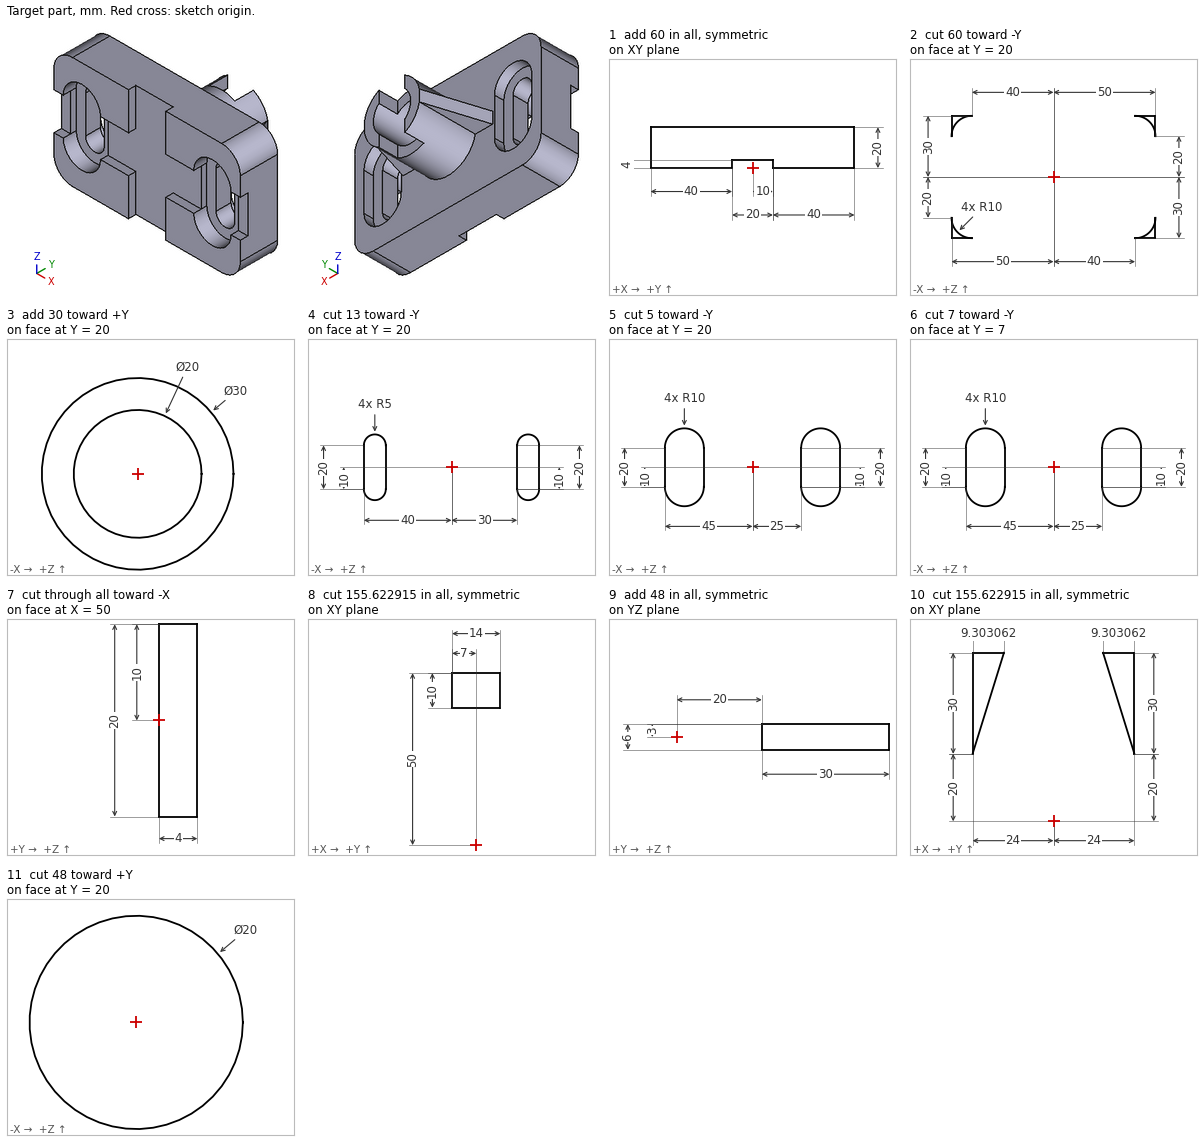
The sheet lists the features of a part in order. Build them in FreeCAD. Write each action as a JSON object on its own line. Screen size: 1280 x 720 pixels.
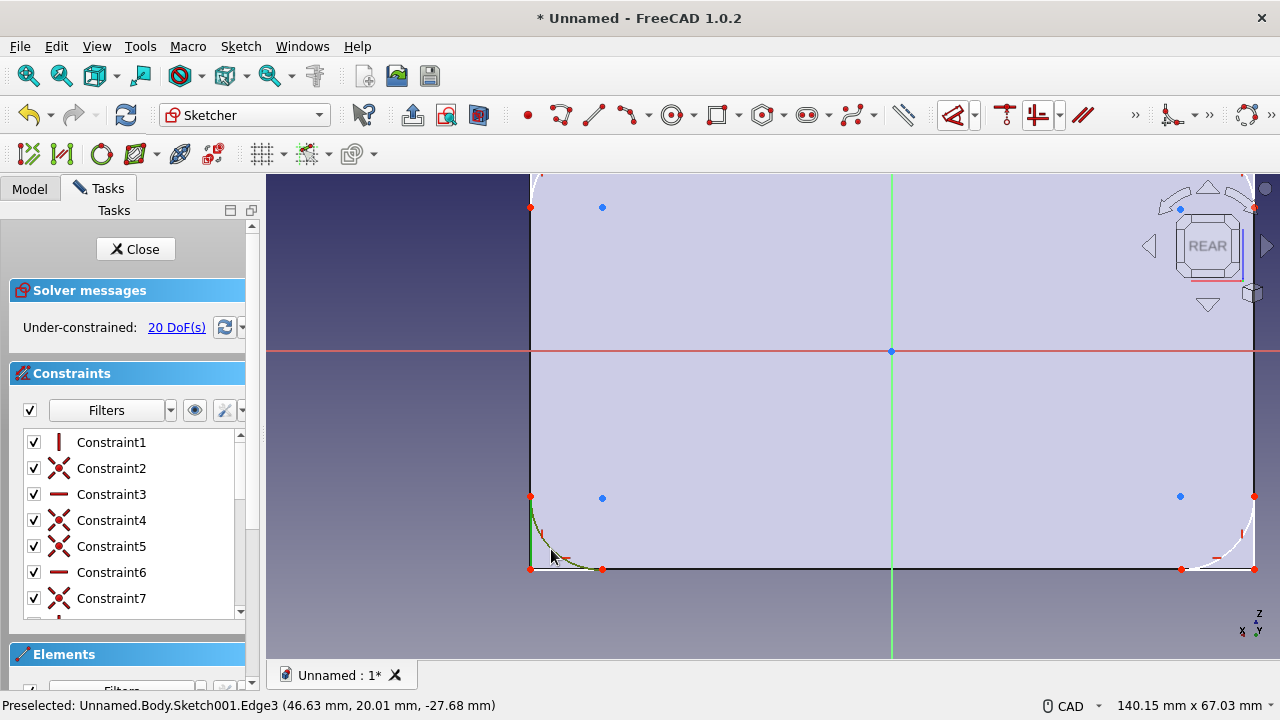
{"action": "key", "text": "t"}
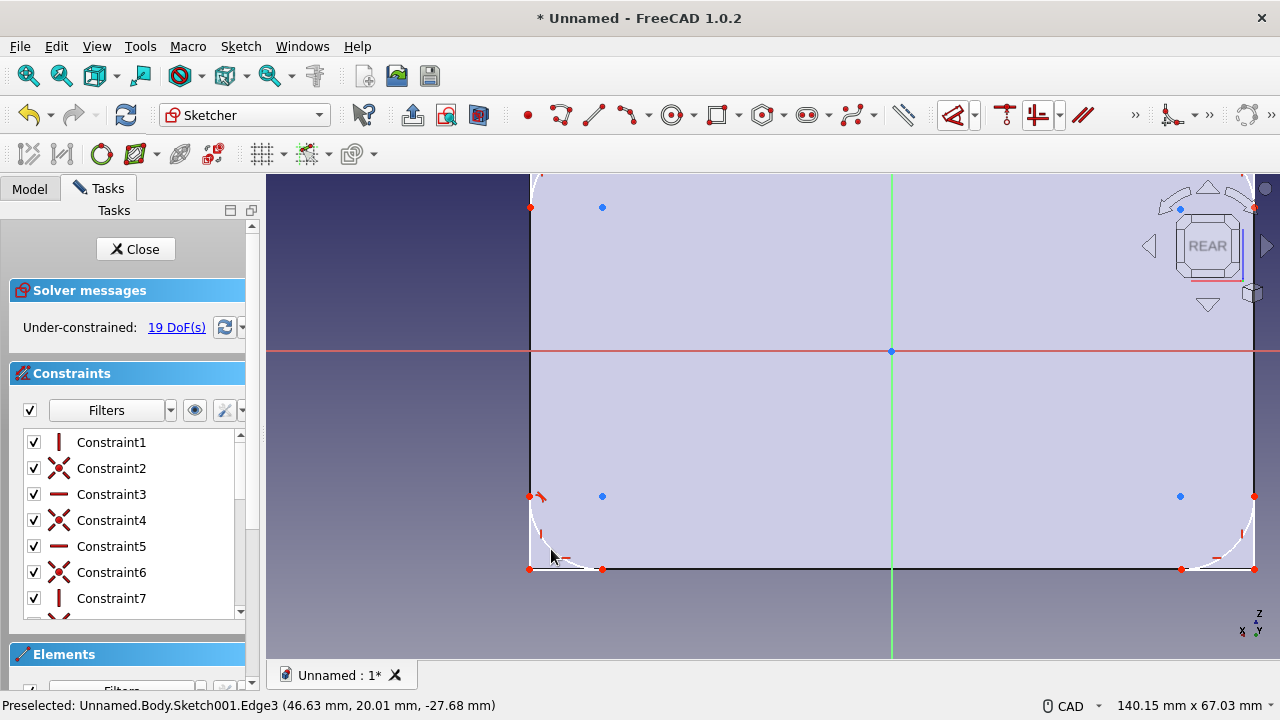
{"action": "left_click", "coordinate": [551, 570]}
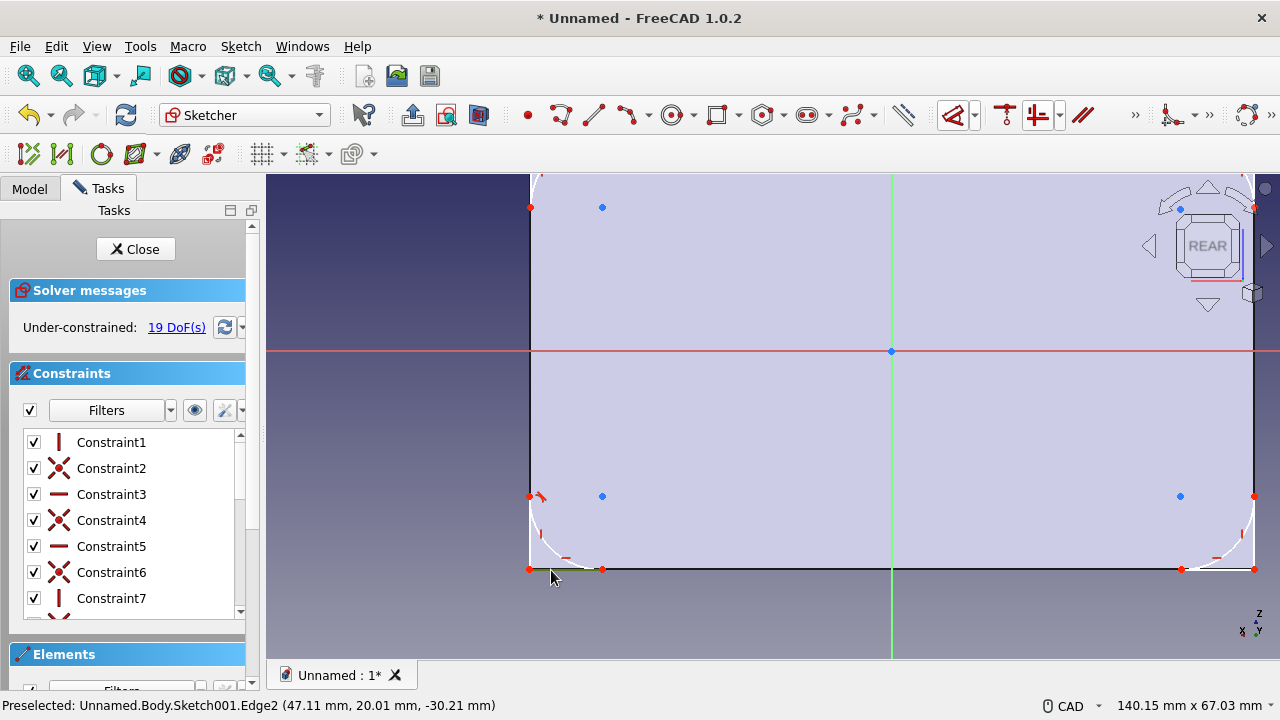
{"action": "left_click", "coordinate": [551, 549]}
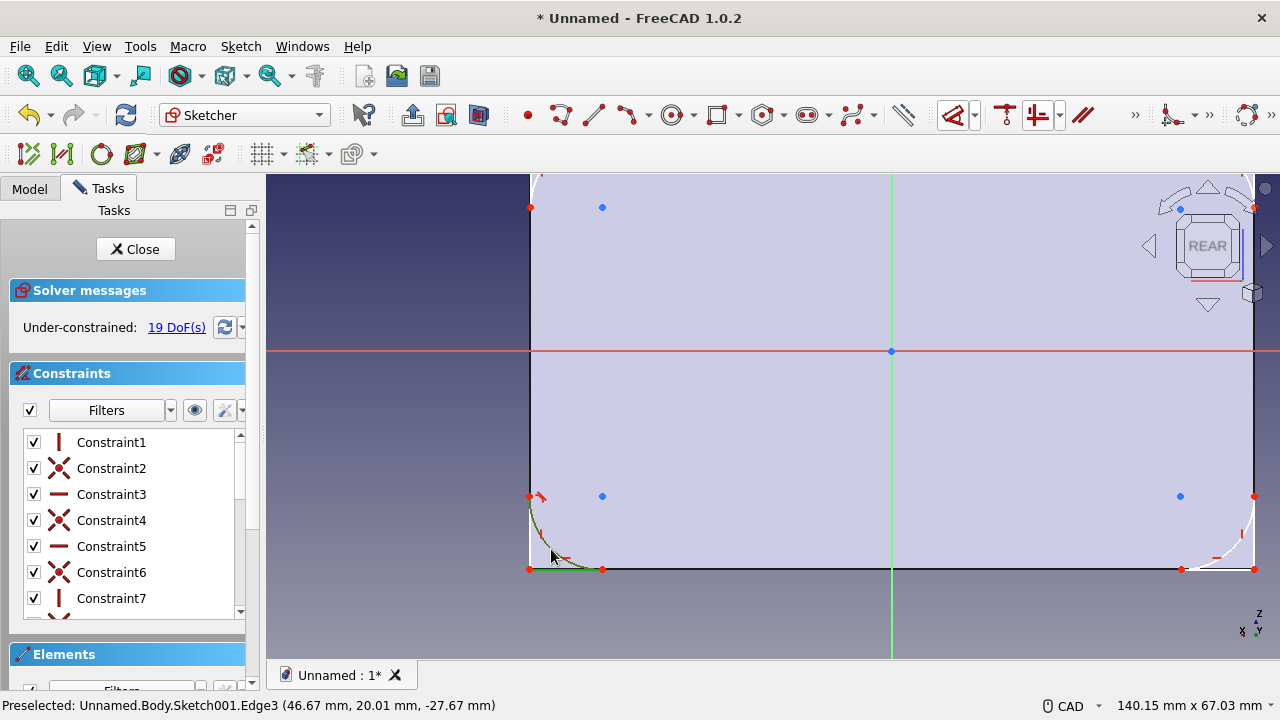
{"action": "key", "text": "t"}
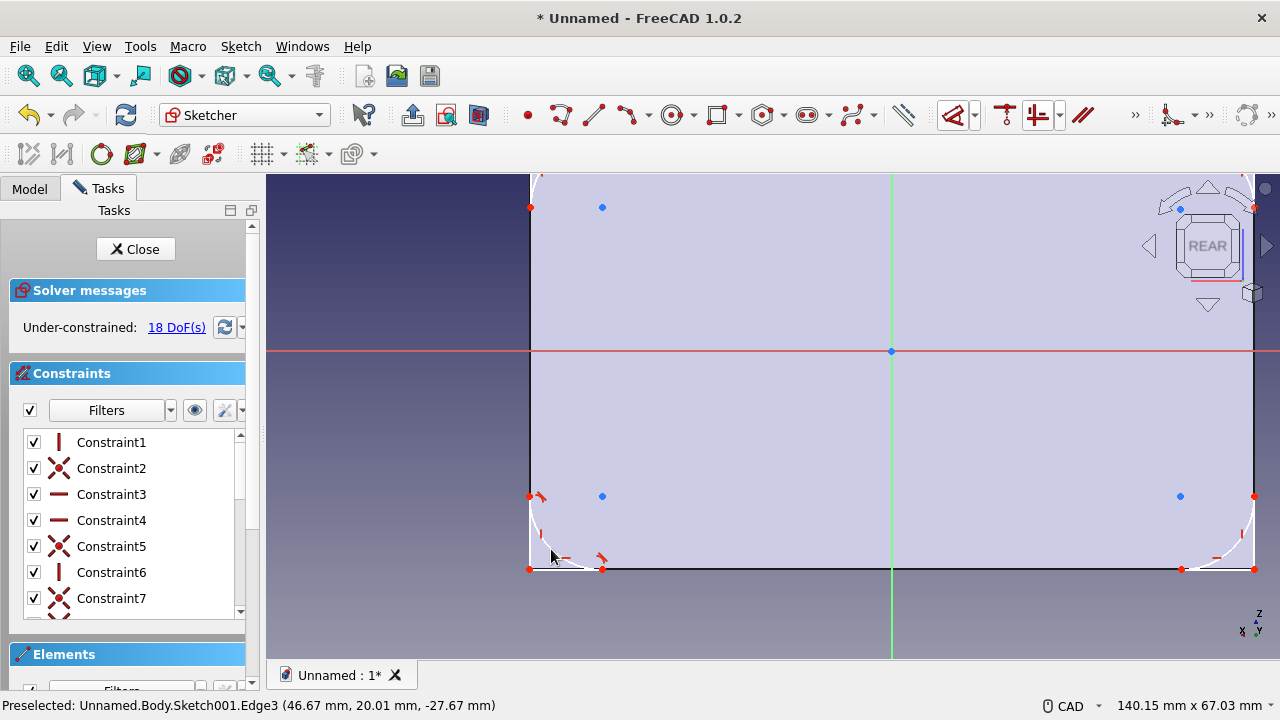
{"action": "scroll", "coordinate": [323, 549], "scroll_direction": "down", "scroll_amount": 2}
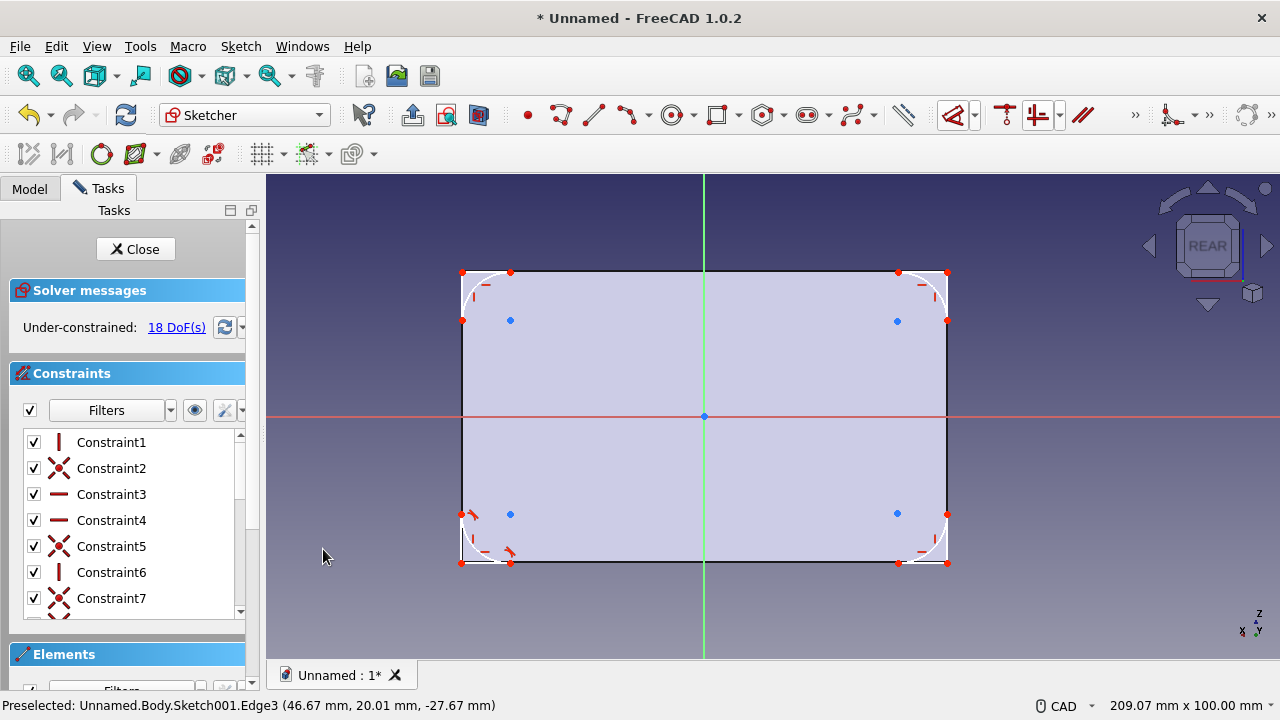
{"action": "scroll", "coordinate": [933, 563], "scroll_direction": "up", "scroll_amount": 2}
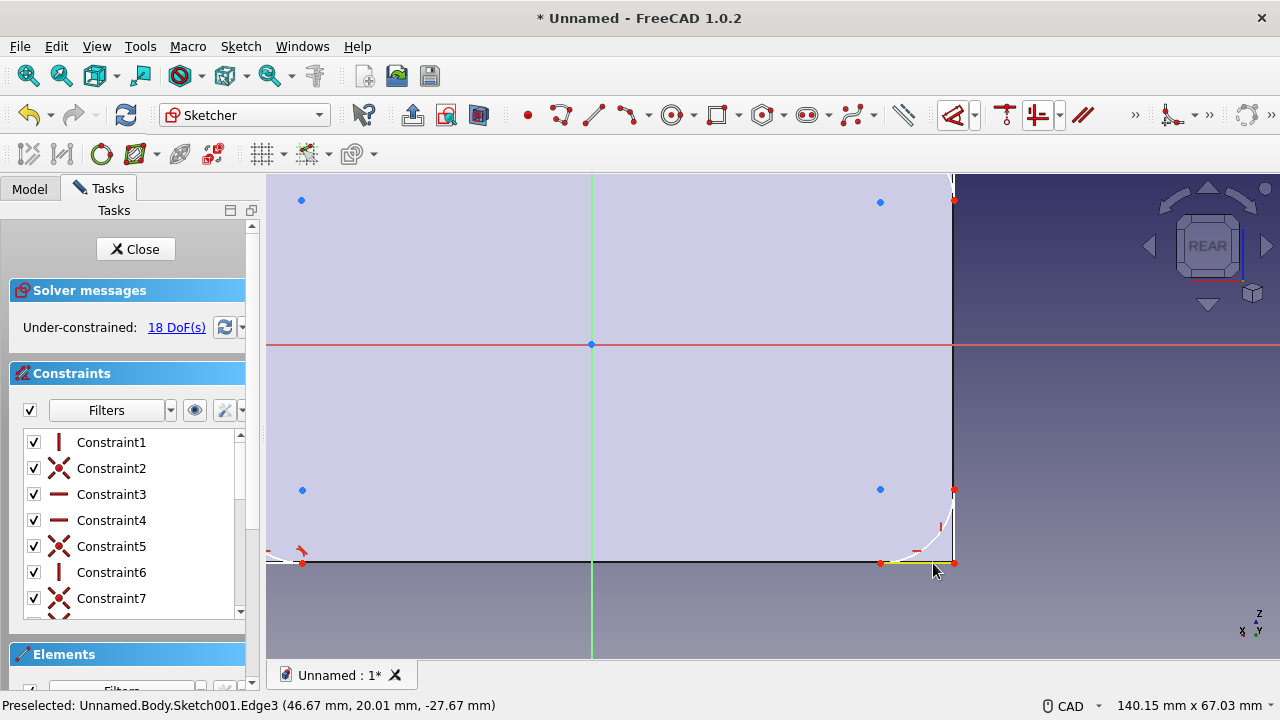
{"action": "left_click", "coordinate": [932, 563]}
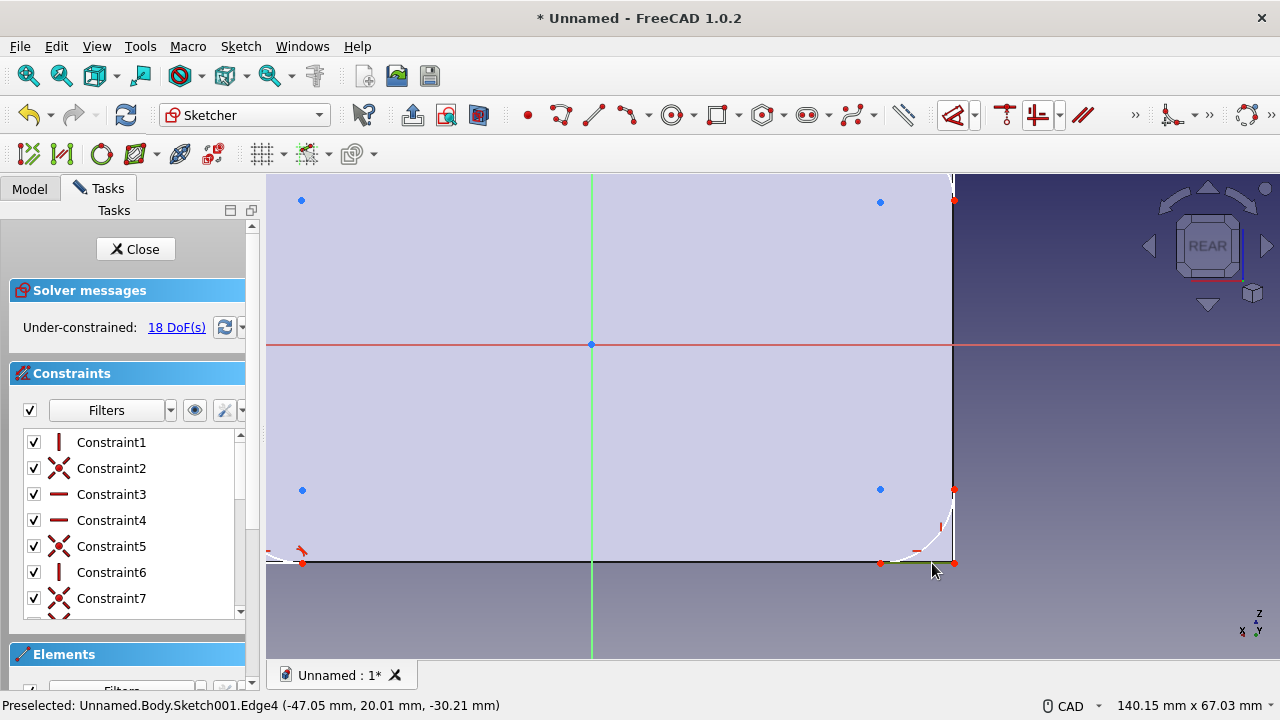
{"action": "left_click", "coordinate": [932, 541]}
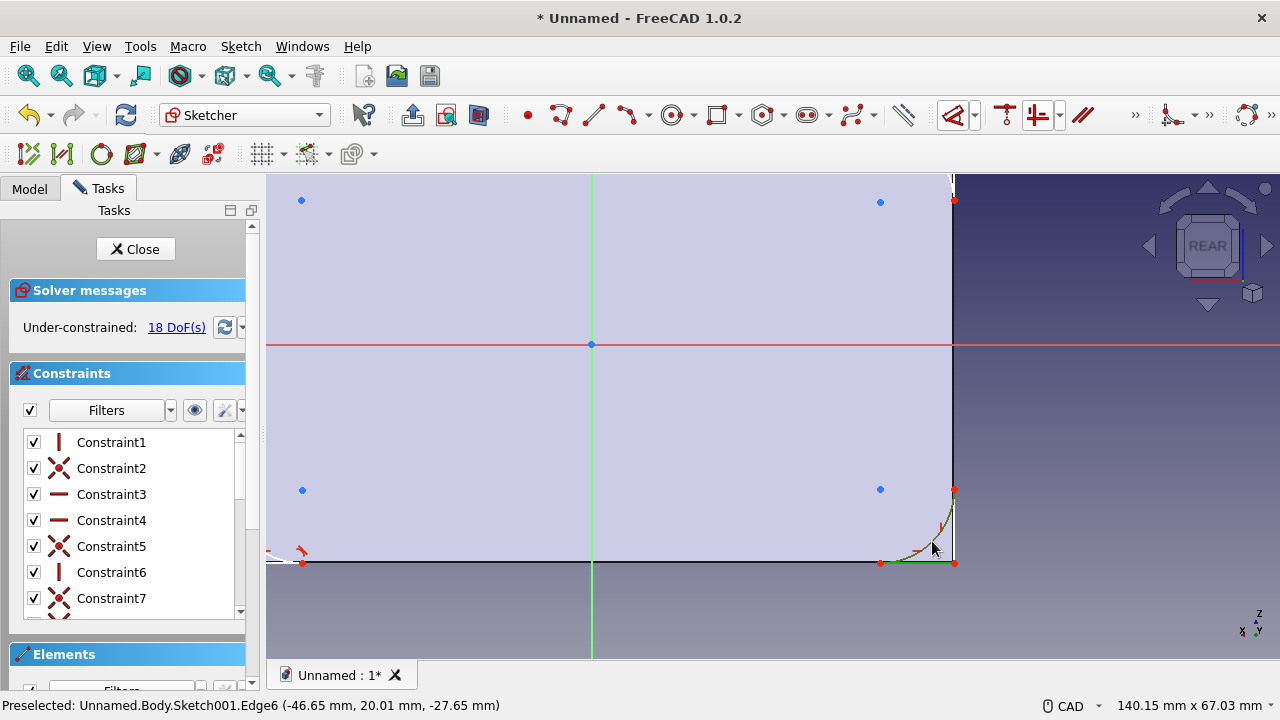
{"action": "key", "text": "t"}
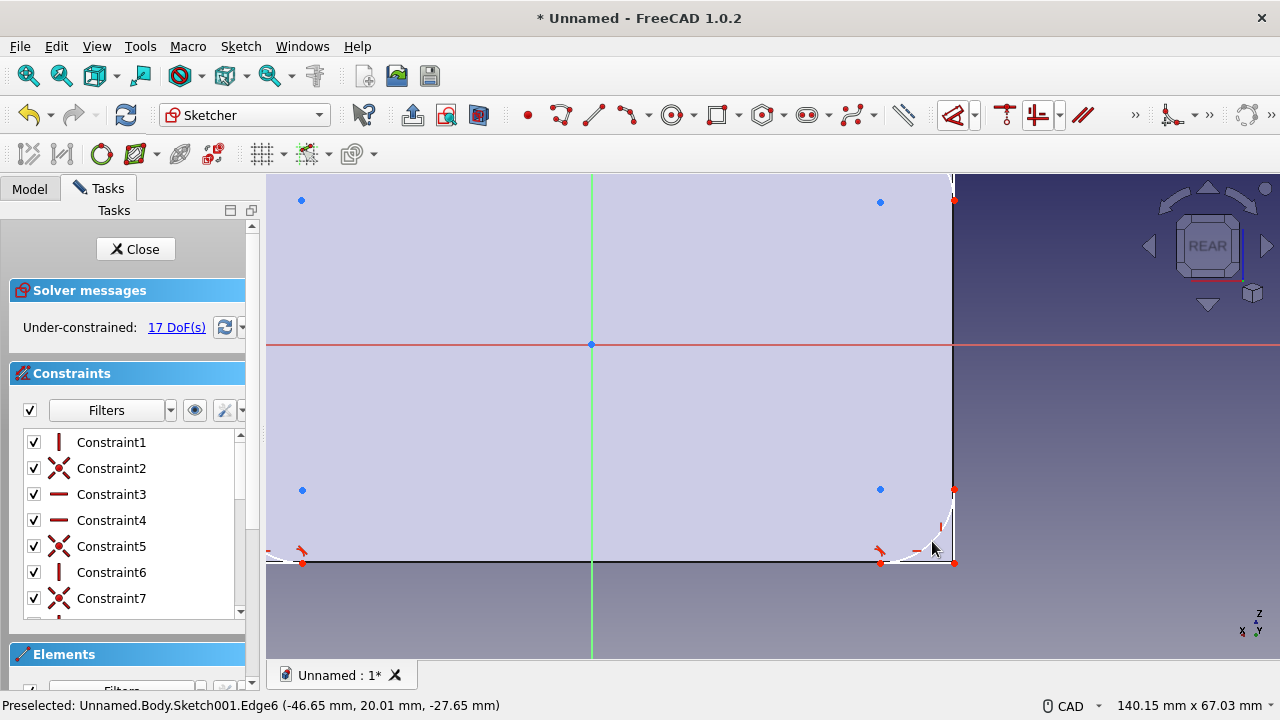
{"action": "left_click", "coordinate": [954, 541]}